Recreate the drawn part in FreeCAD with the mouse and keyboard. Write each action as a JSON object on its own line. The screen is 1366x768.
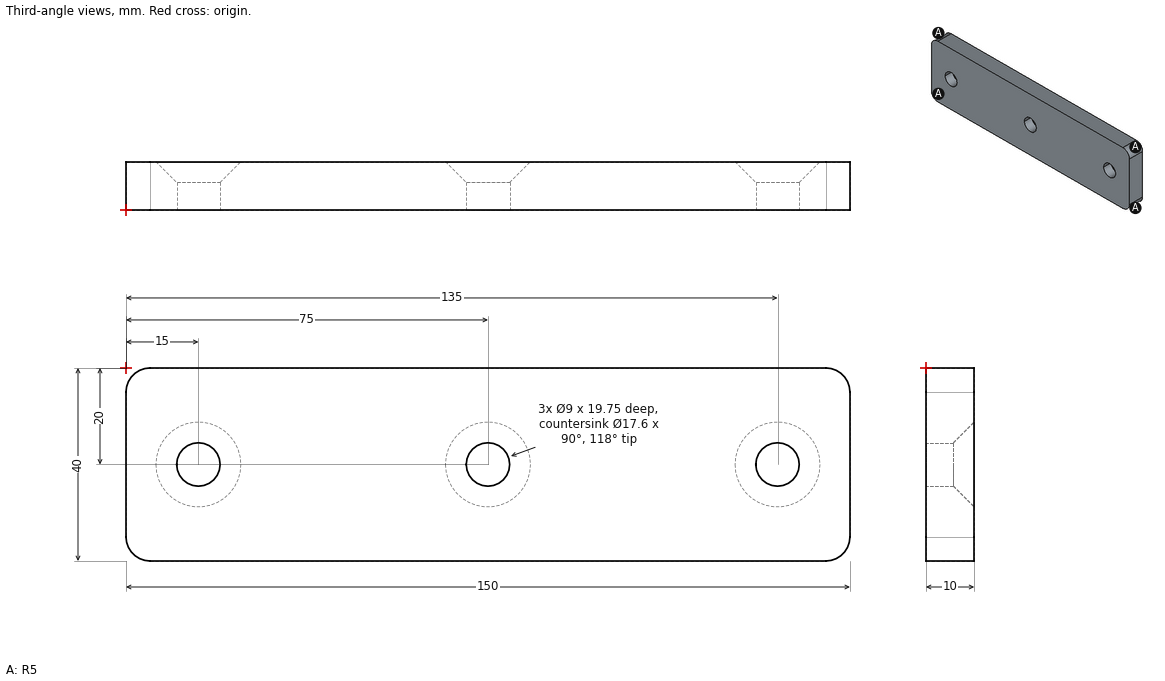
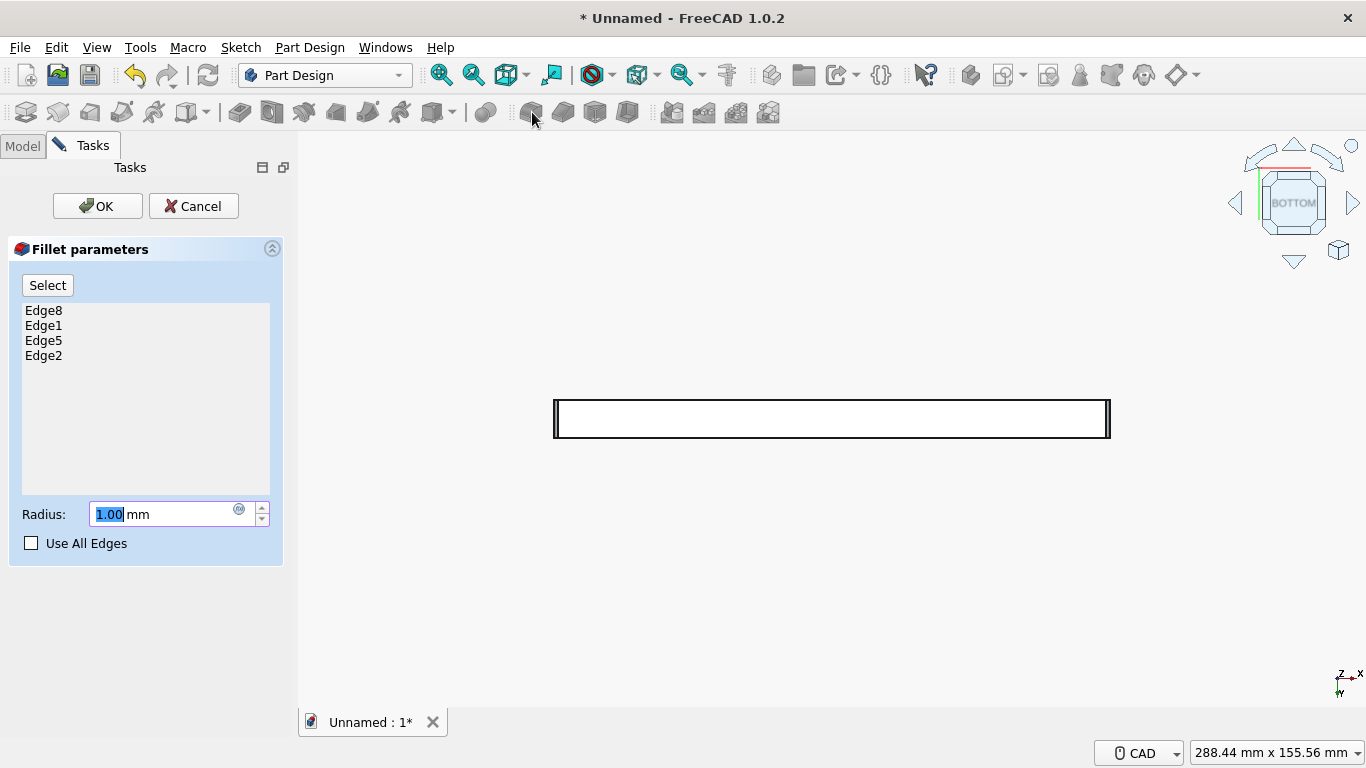
{"action": "type", "text": "5"}
{"action": "key", "text": "Tab"}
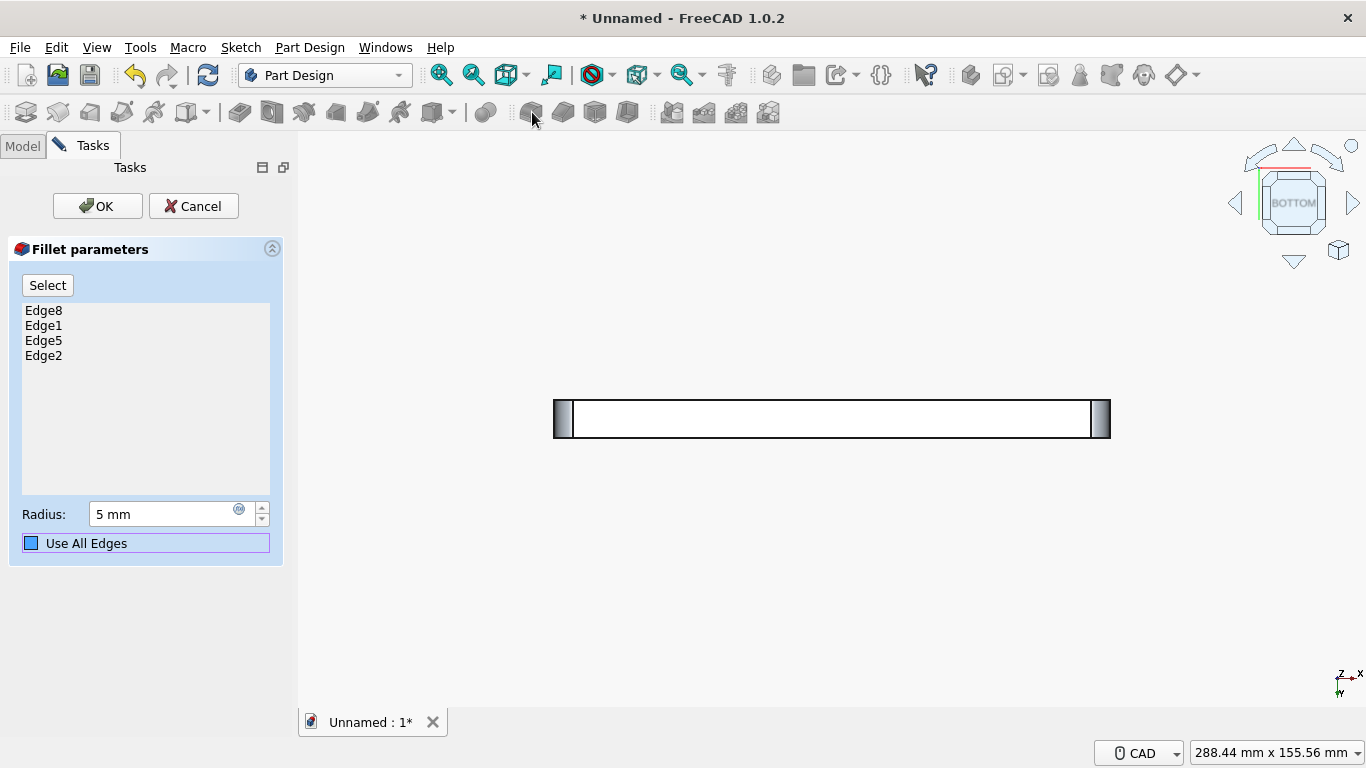
{"action": "left_click", "coordinate": [98, 206]}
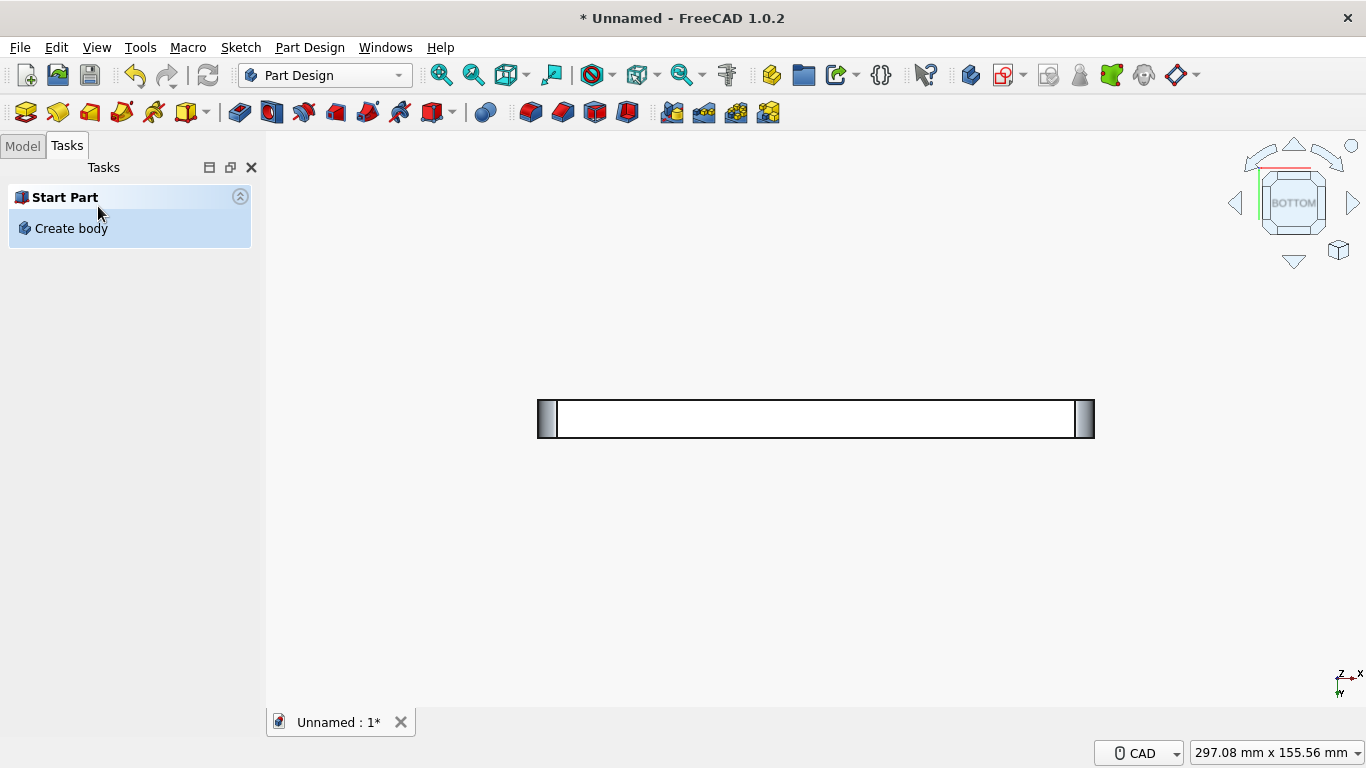
{"action": "key", "text": "4"}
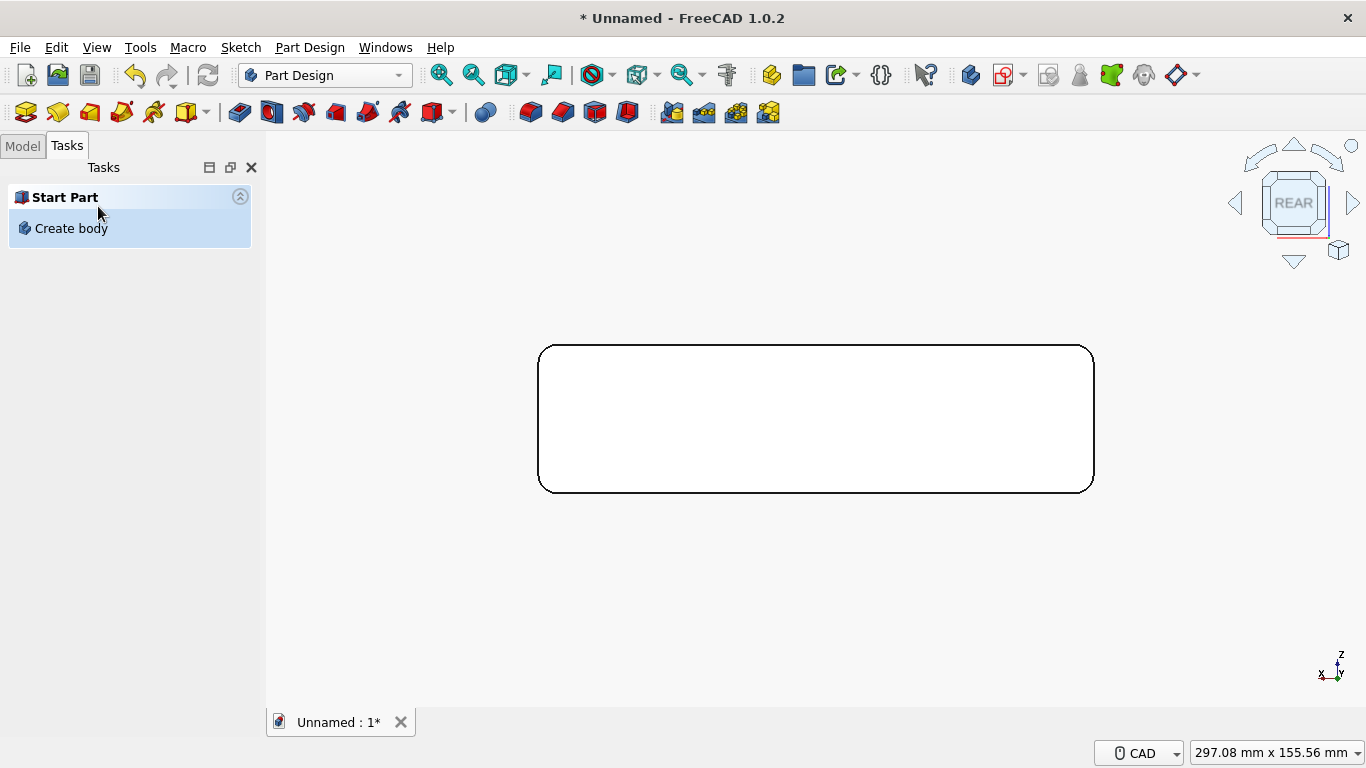
{"action": "left_click", "coordinate": [657, 418]}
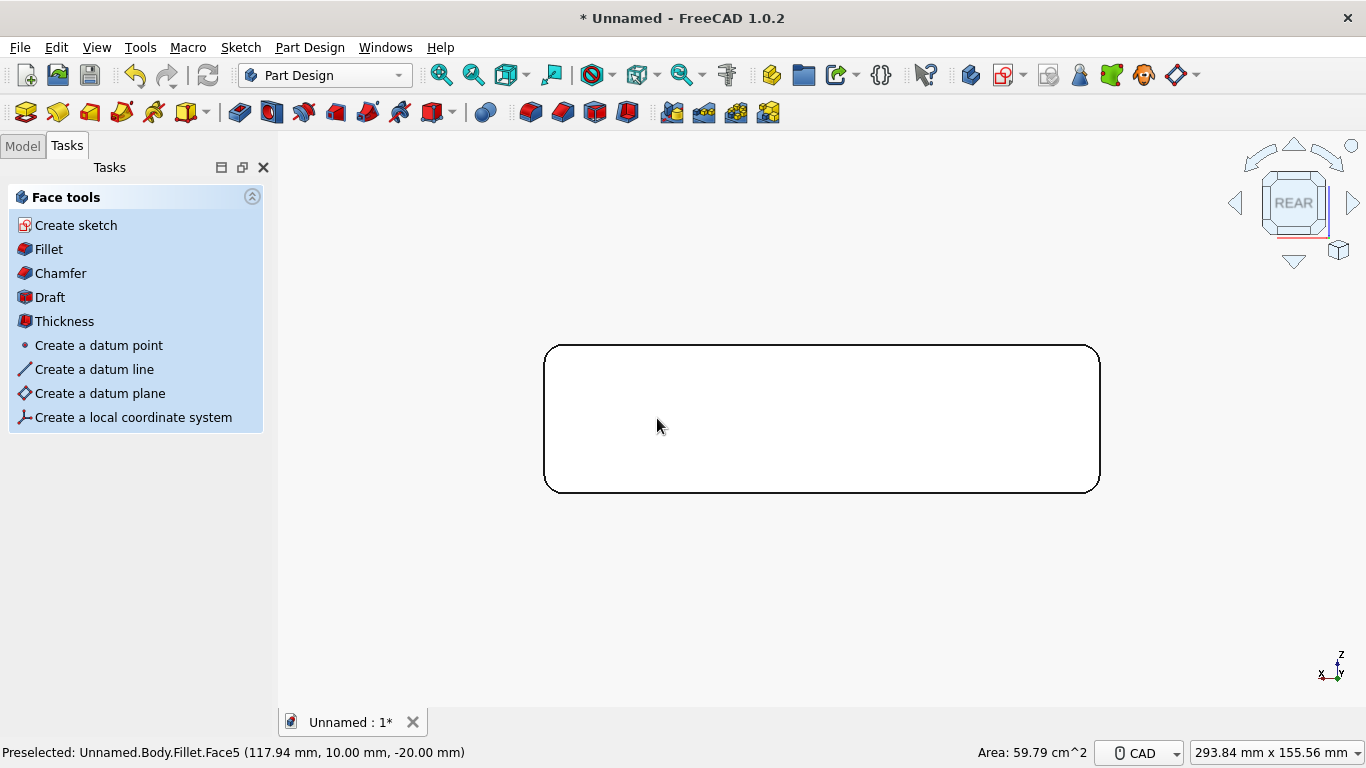
{"action": "left_click", "coordinate": [1004, 76]}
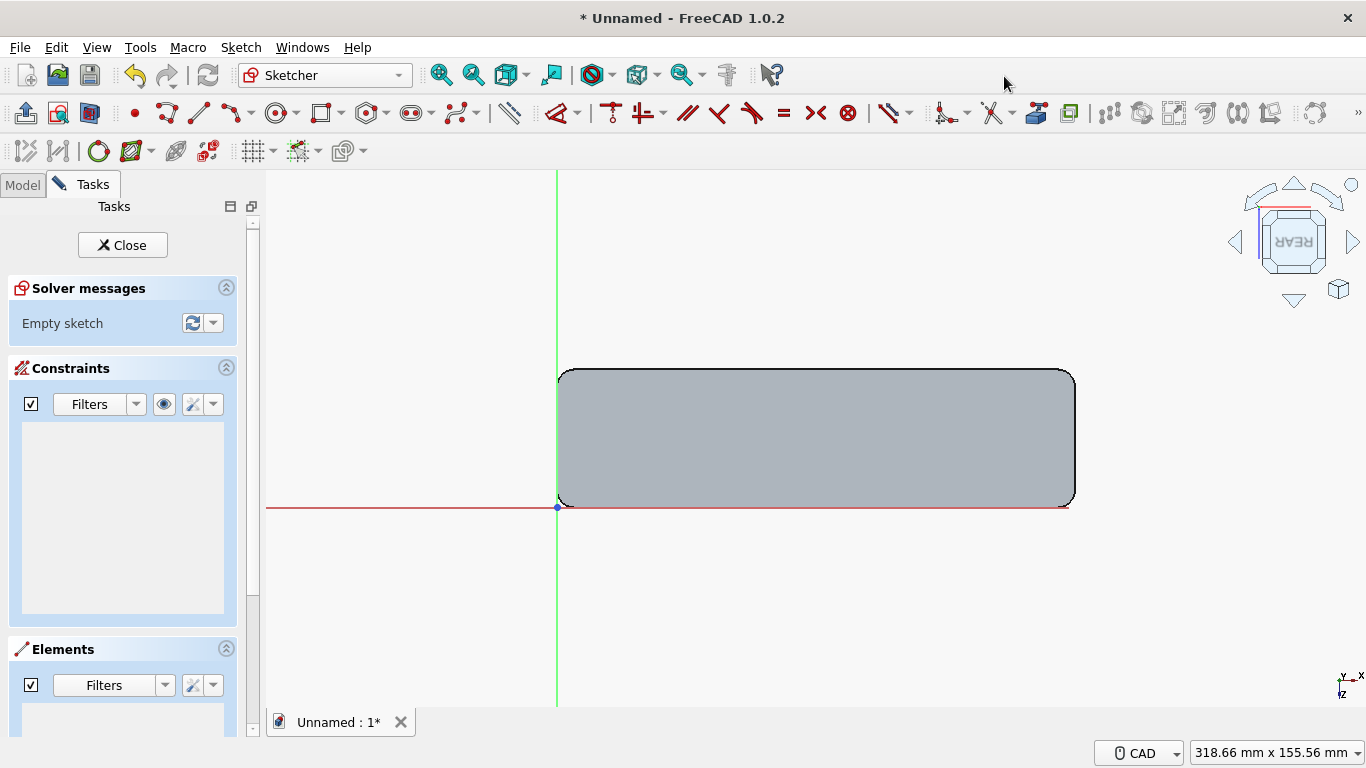
{"action": "left_click", "coordinate": [276, 114]}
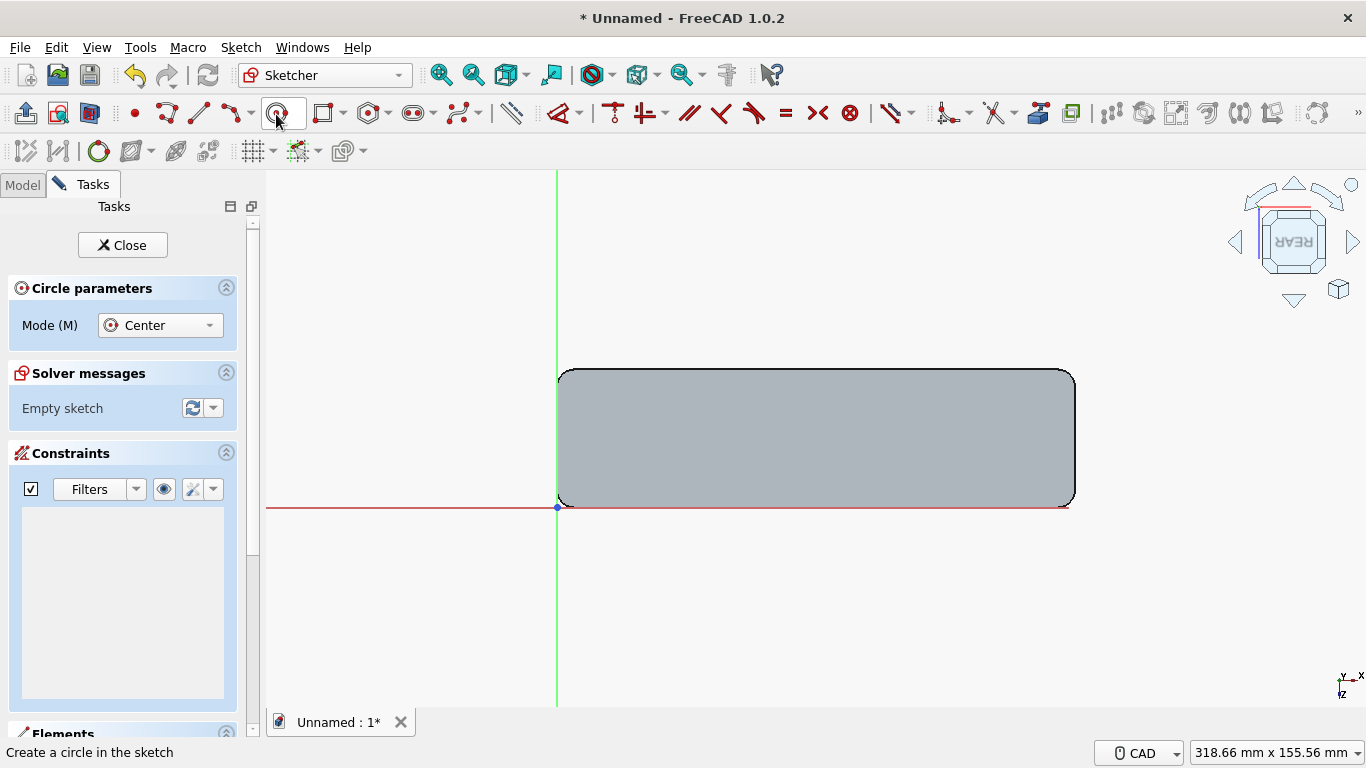
{"action": "scroll", "coordinate": [816, 439], "scroll_direction": "up", "scroll_amount": 2}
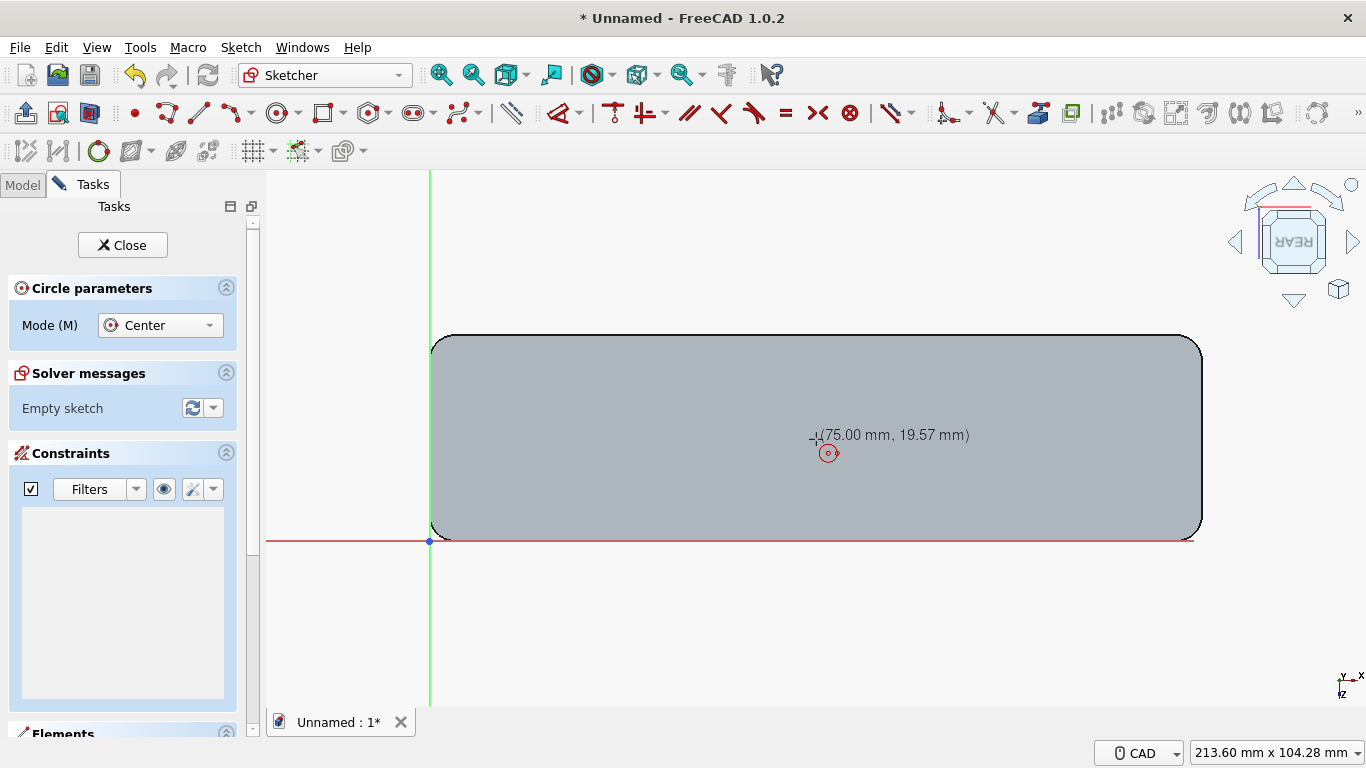
{"action": "left_click", "coordinate": [816, 438]}
{"action": "left_click", "coordinate": [832, 422]}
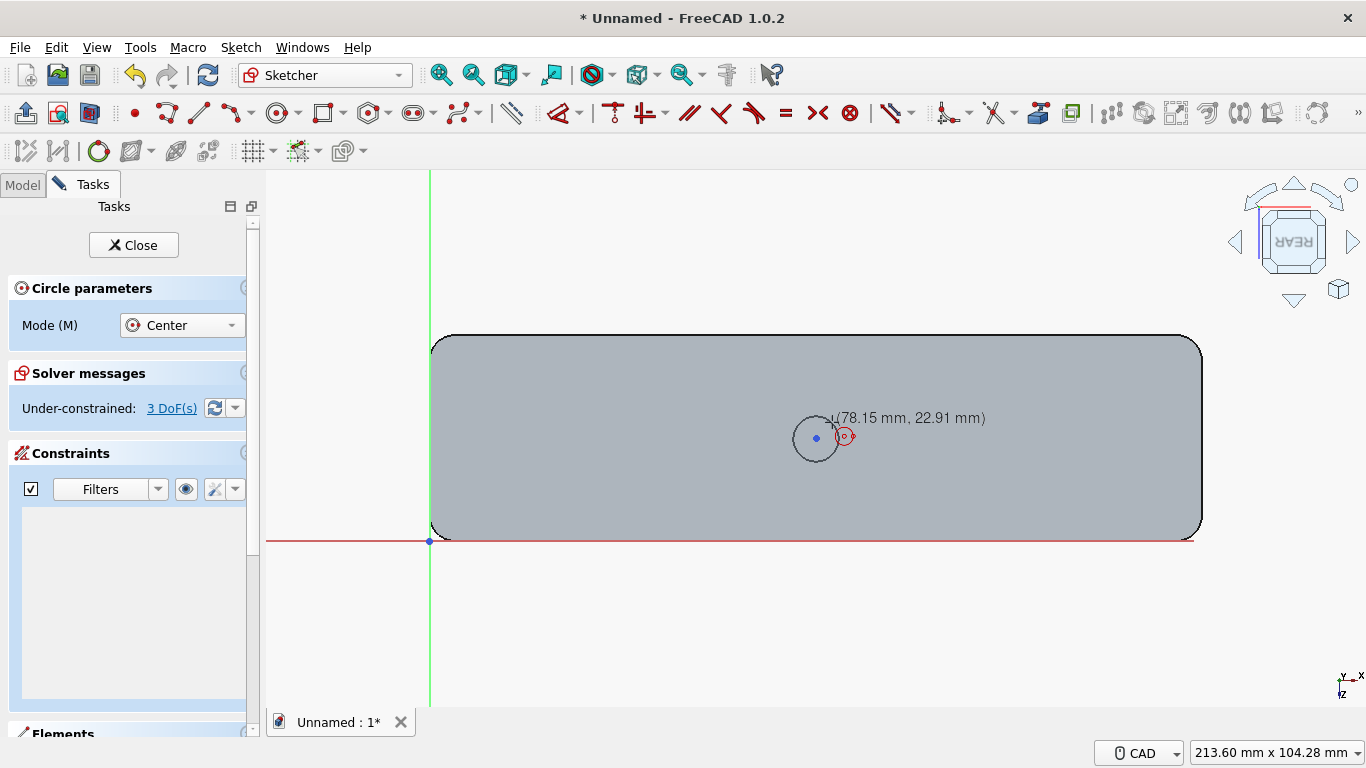
{"action": "left_click", "coordinate": [507, 438]}
{"action": "left_click", "coordinate": [523, 422]}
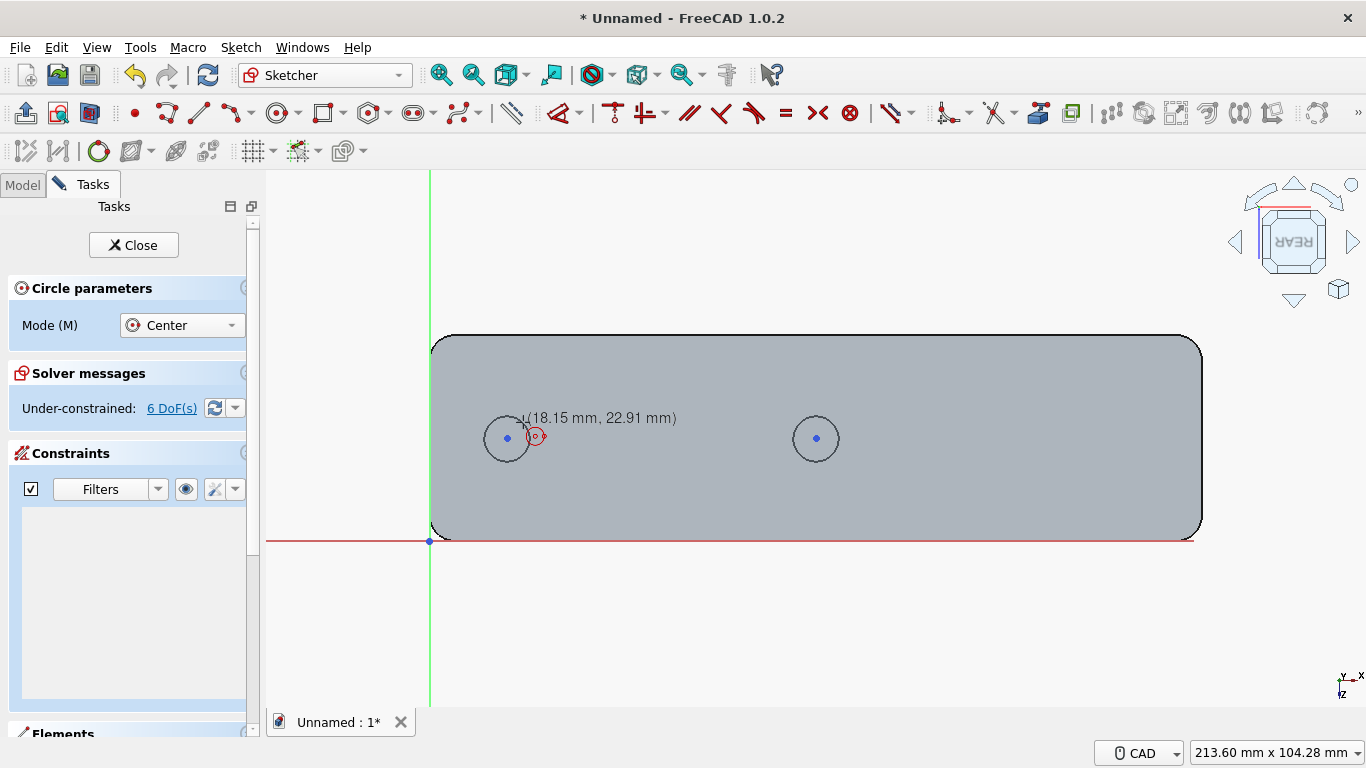
{"action": "left_click", "coordinate": [1125, 438]}
{"action": "left_click", "coordinate": [1141, 422]}
{"action": "key", "text": "Escape"}